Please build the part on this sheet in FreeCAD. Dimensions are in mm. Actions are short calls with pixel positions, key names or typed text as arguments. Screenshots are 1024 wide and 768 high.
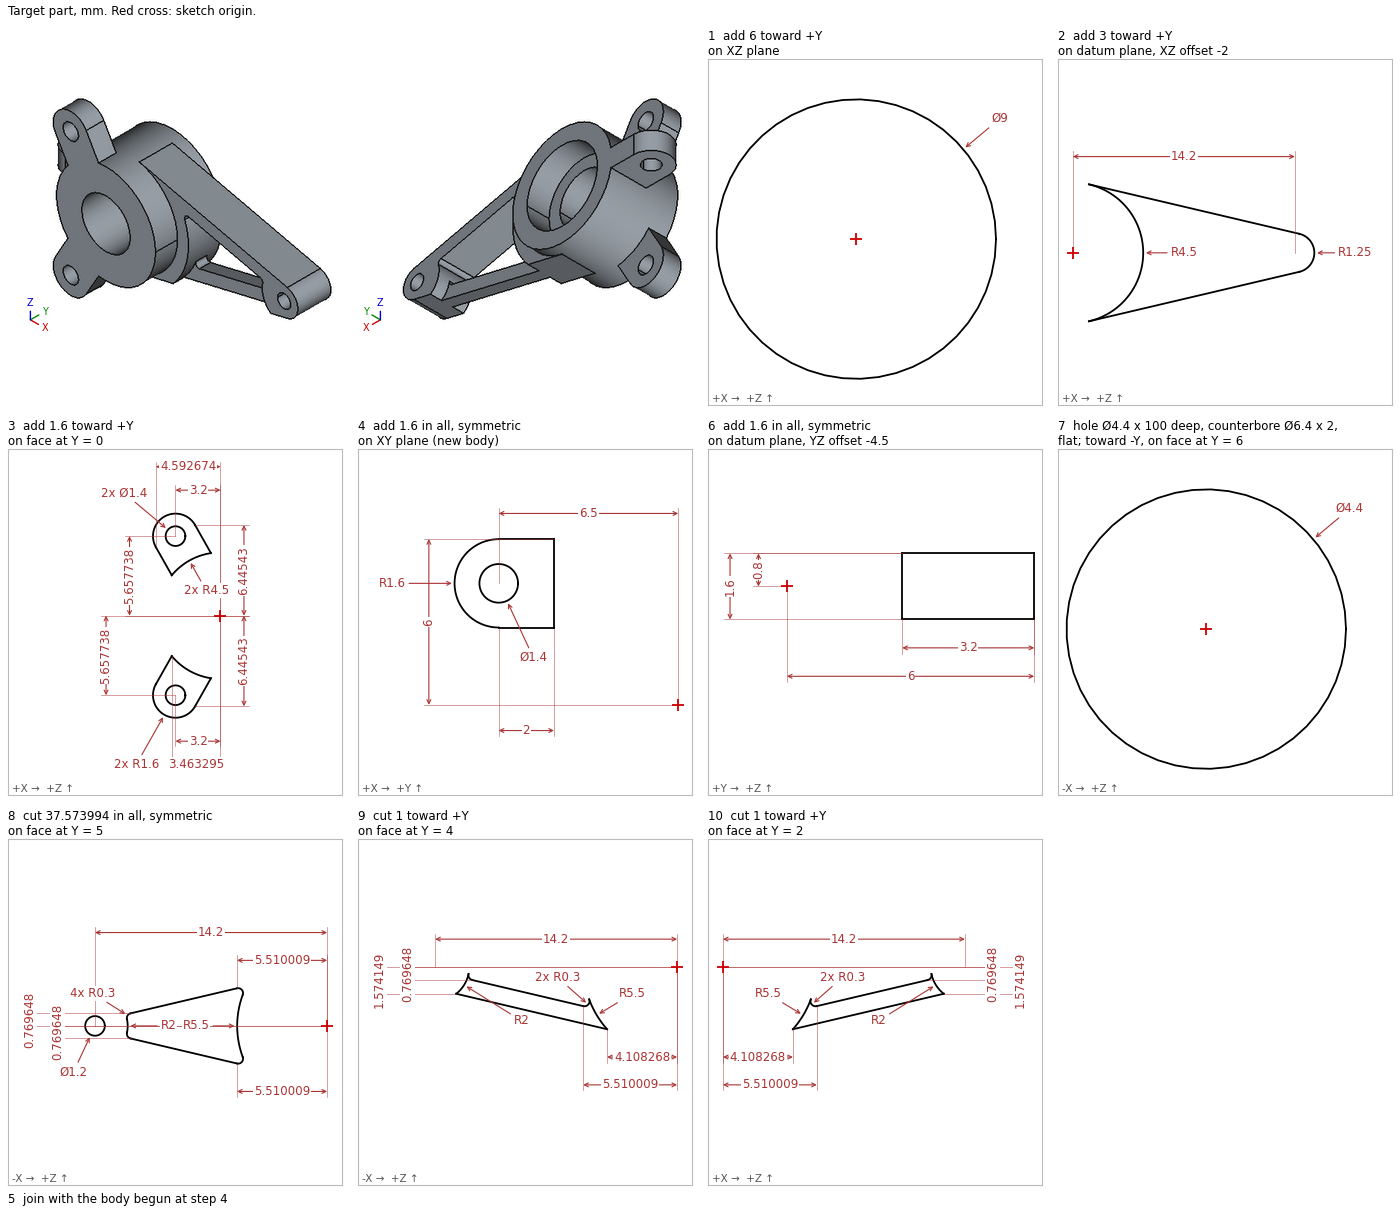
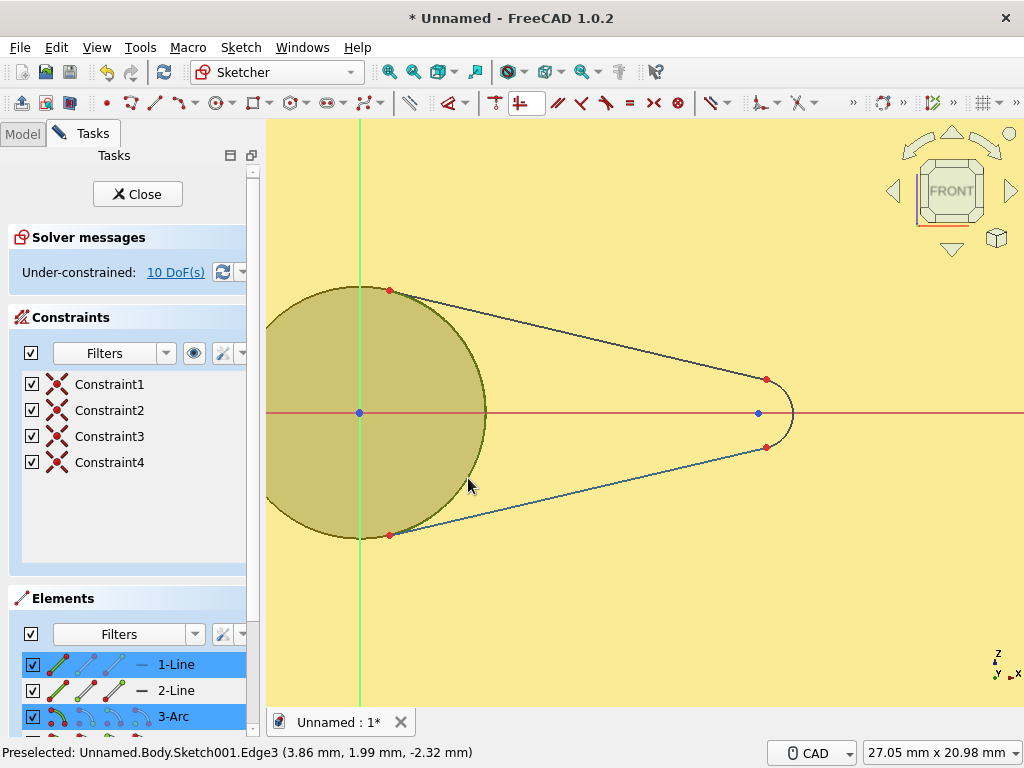
key(t)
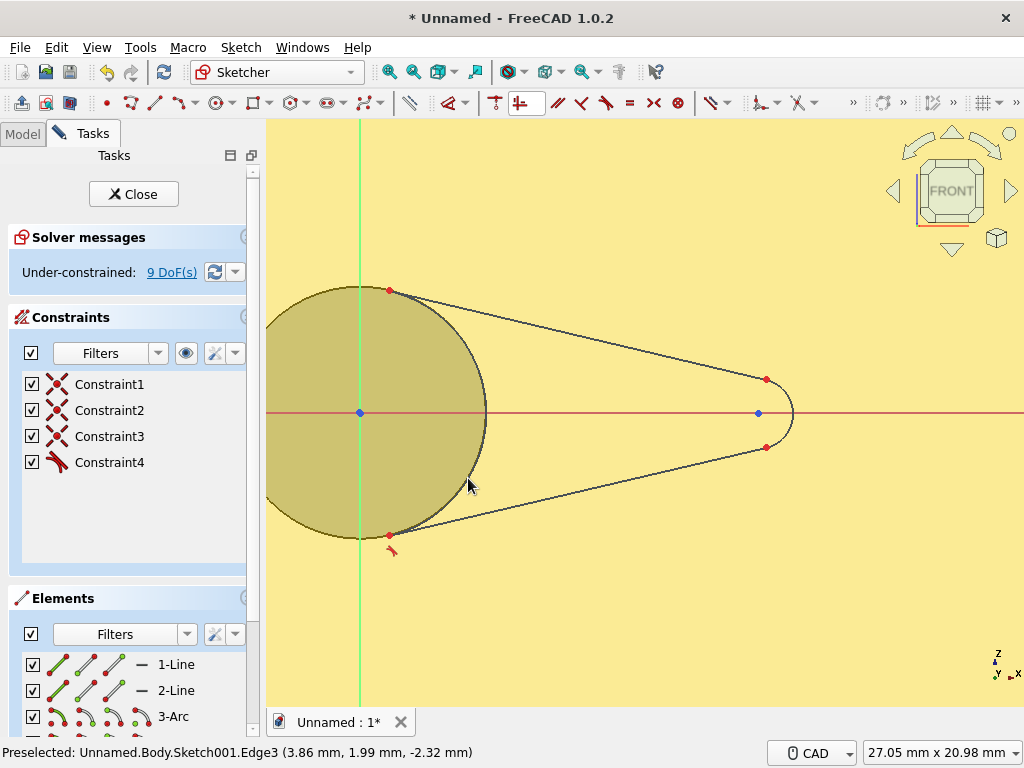
click(653, 474)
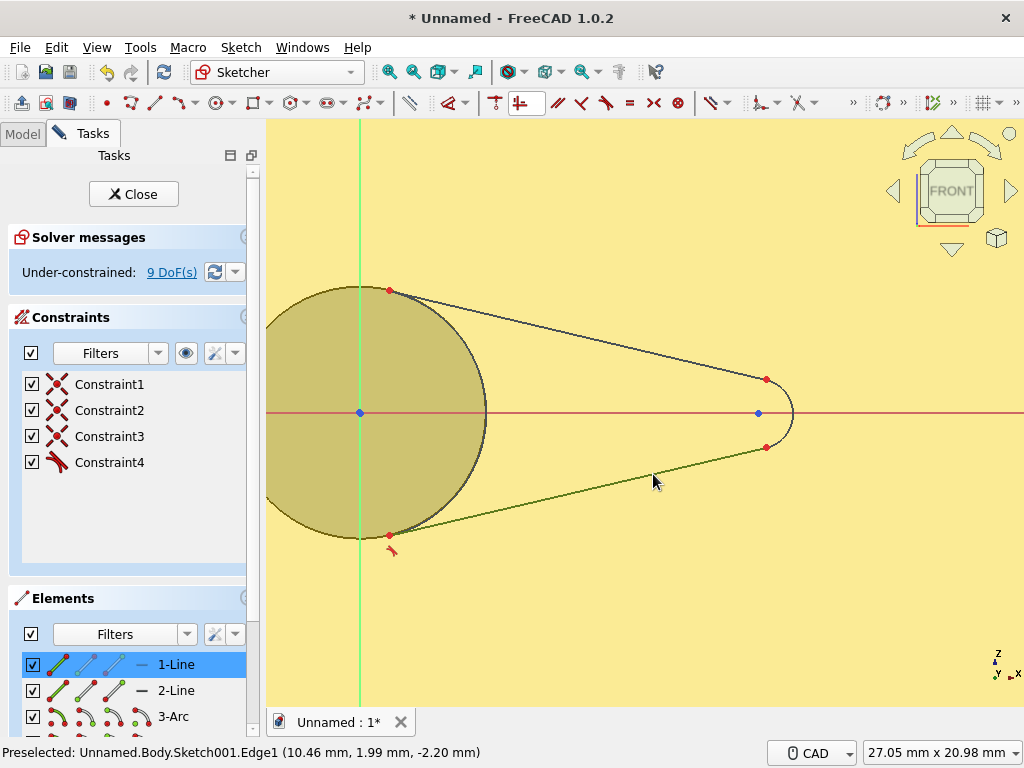
click(788, 432)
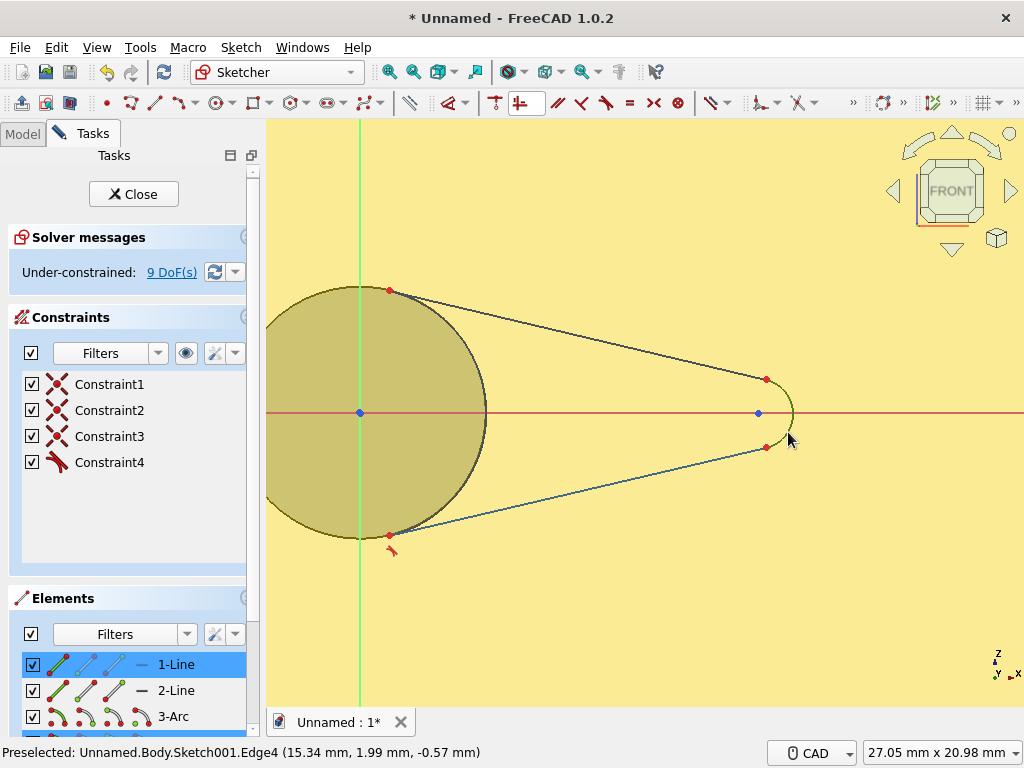
click(606, 104)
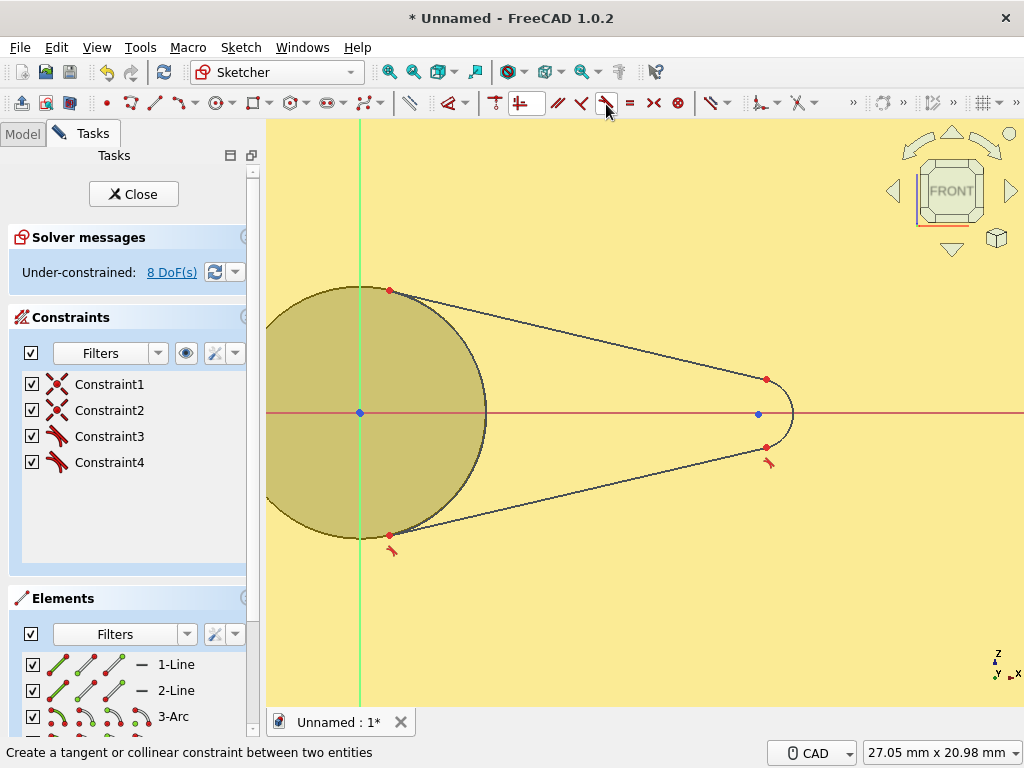
click(502, 318)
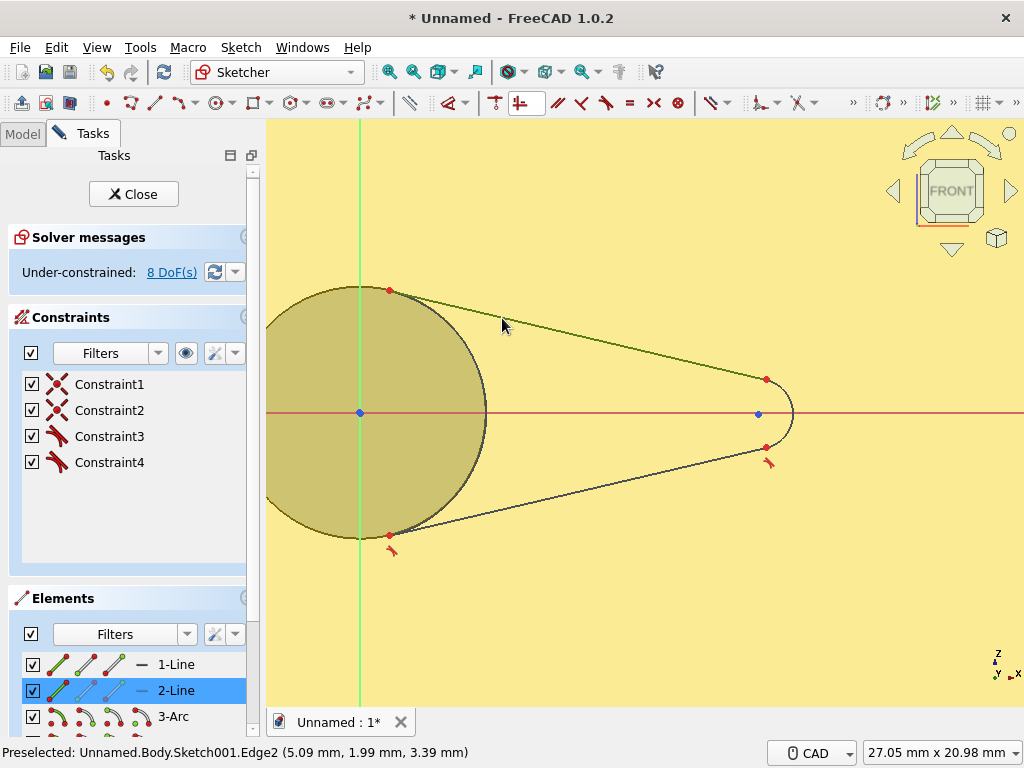
click(469, 478)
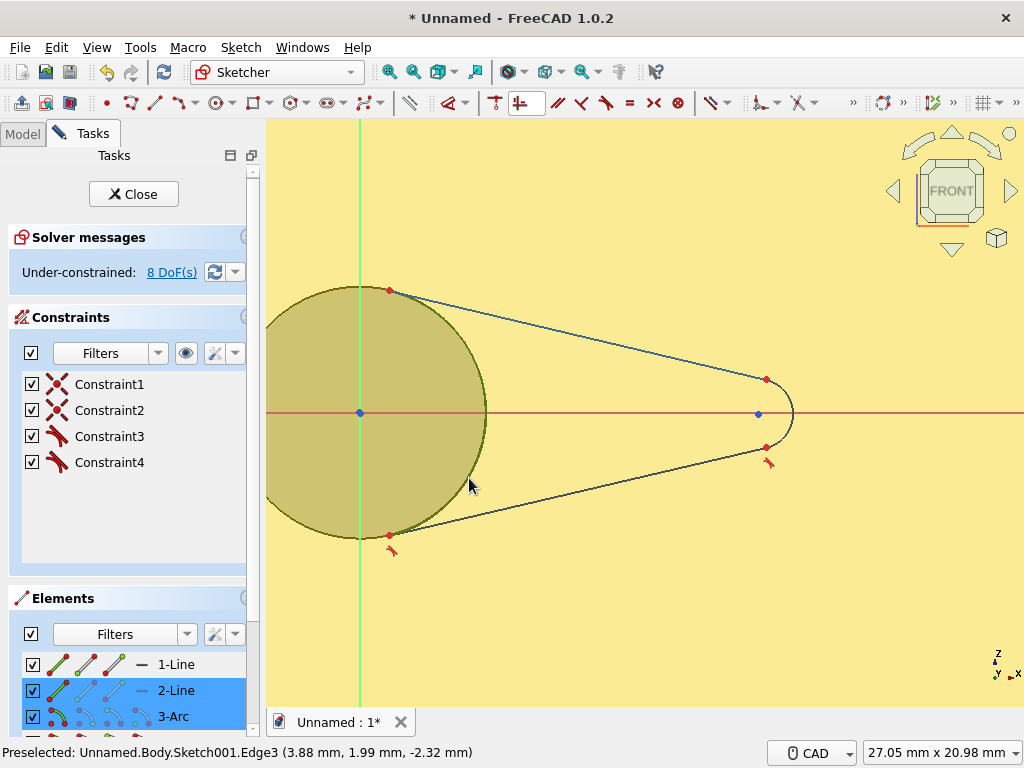
click(606, 104)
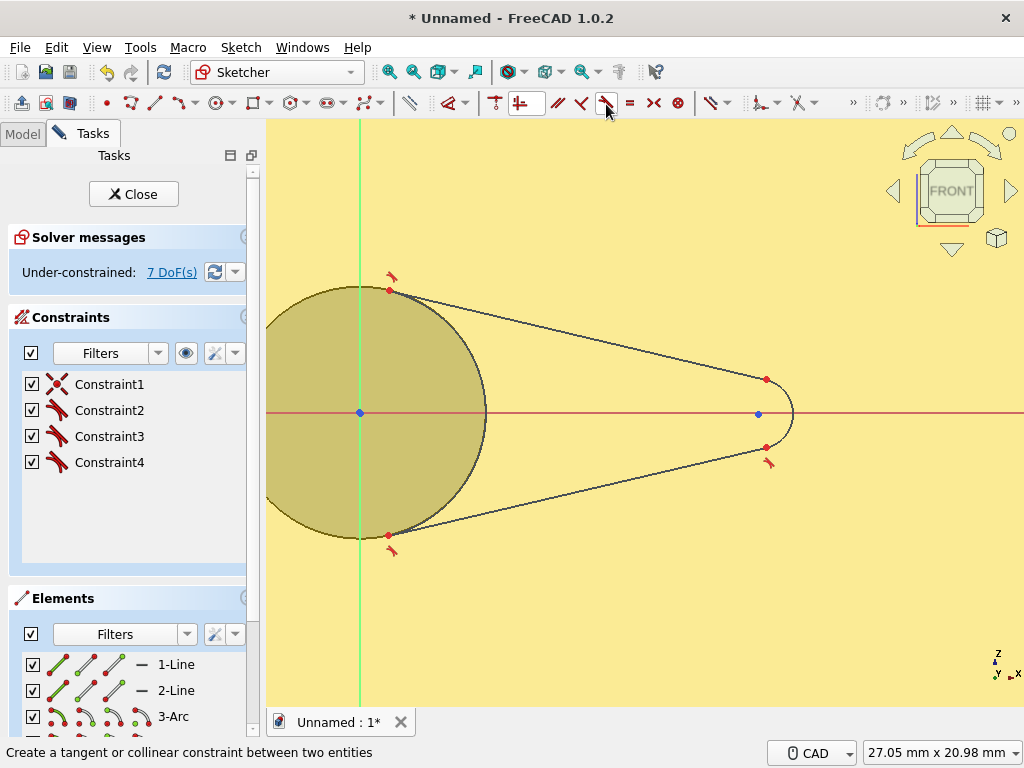
click(502, 318)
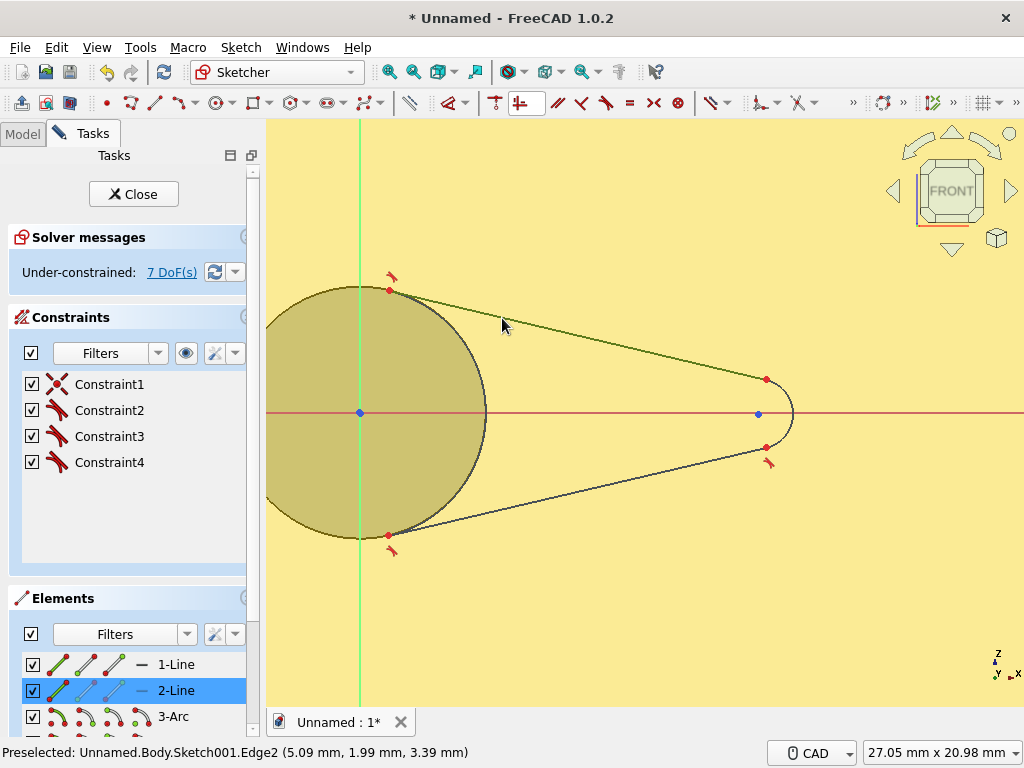
click(788, 432)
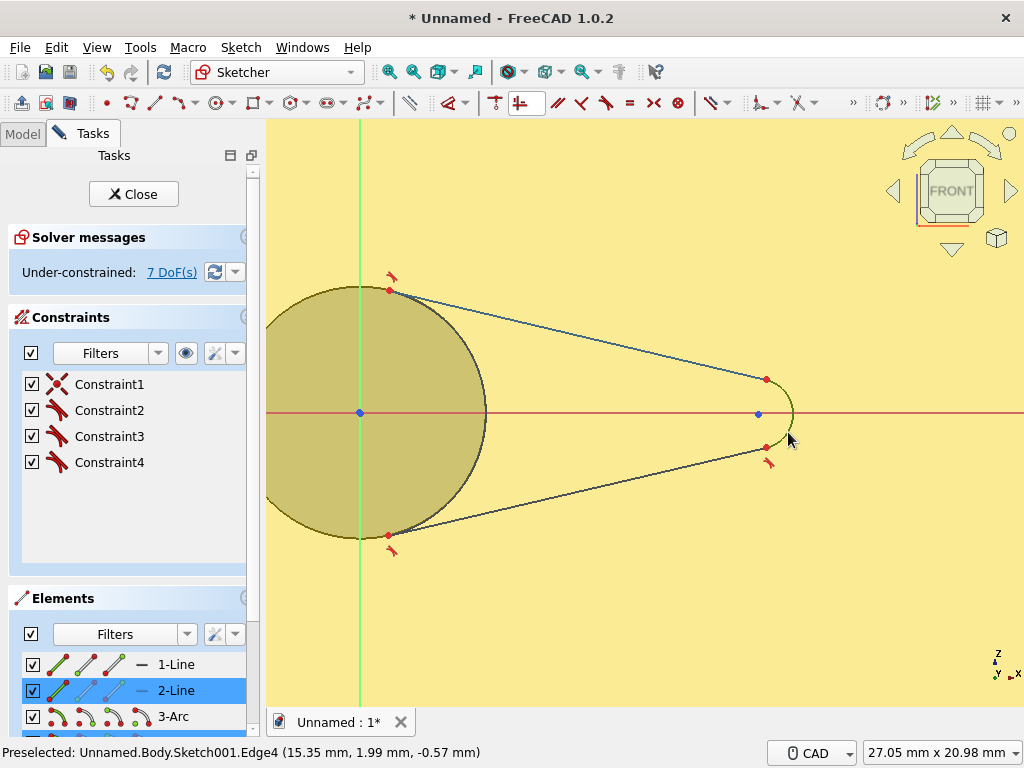
key(t)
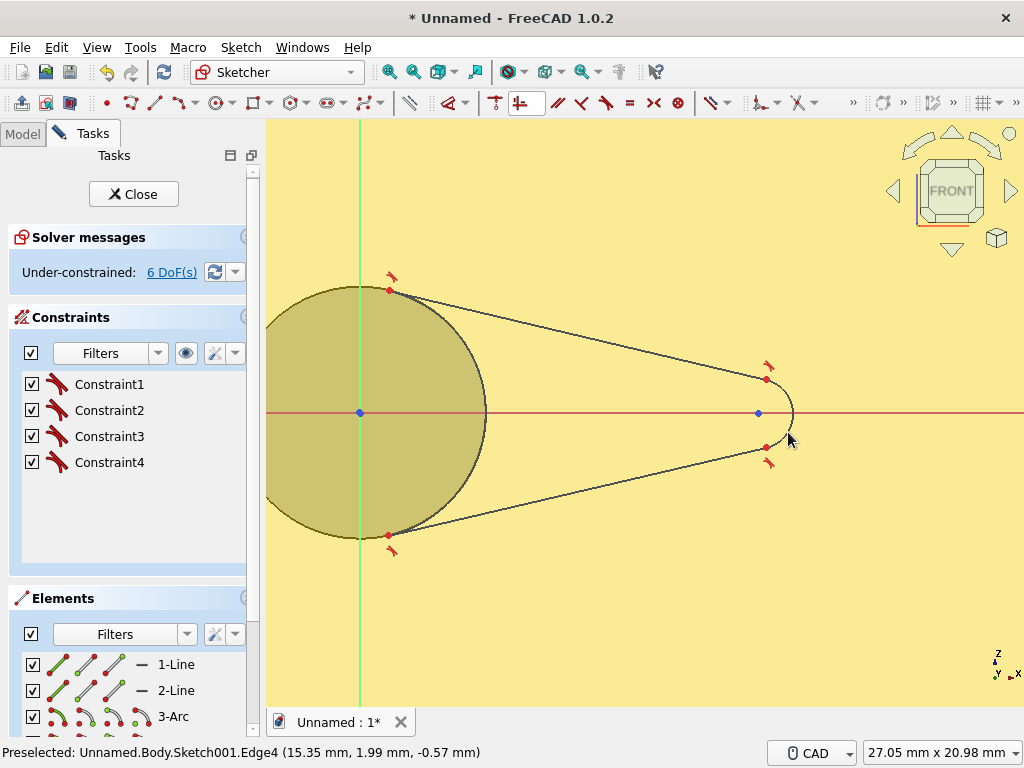
drag(350, 403, 370, 423)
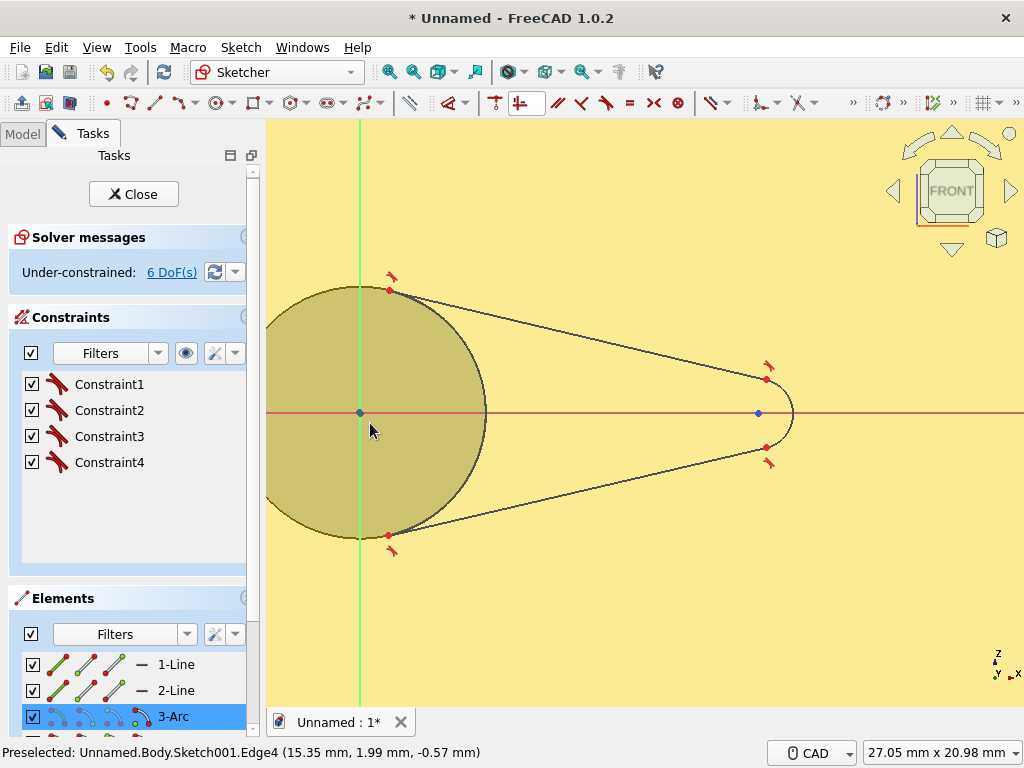
key(c)